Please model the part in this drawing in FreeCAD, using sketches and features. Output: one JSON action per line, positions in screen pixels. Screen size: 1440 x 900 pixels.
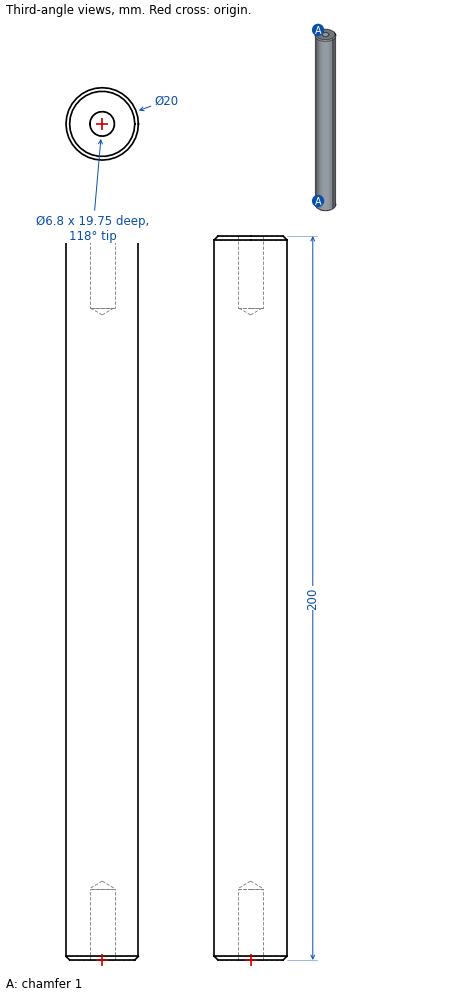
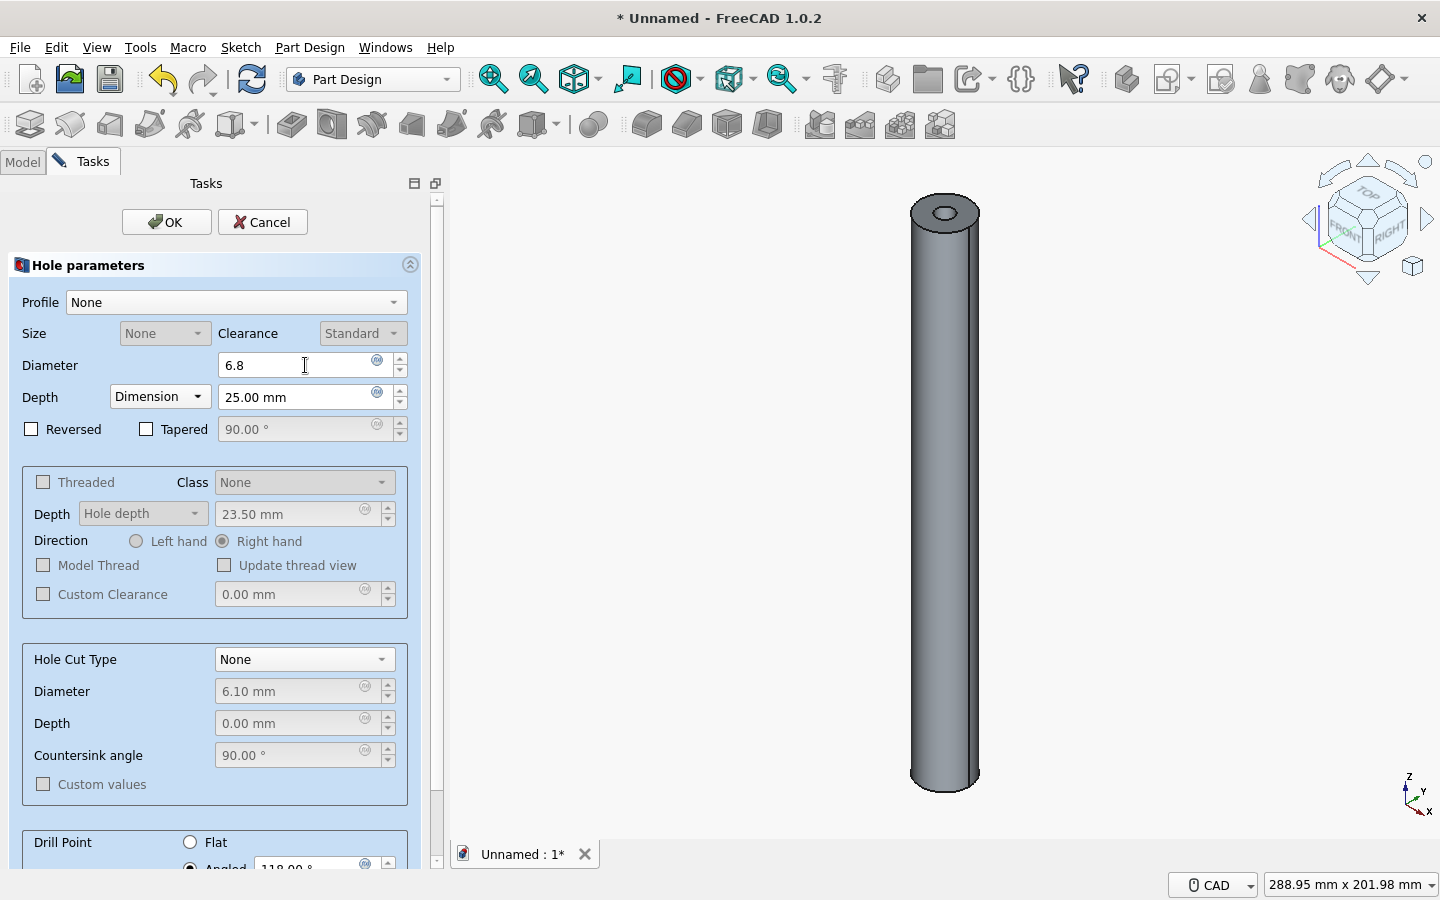
{"action": "triple_click", "coordinate": [305, 397]}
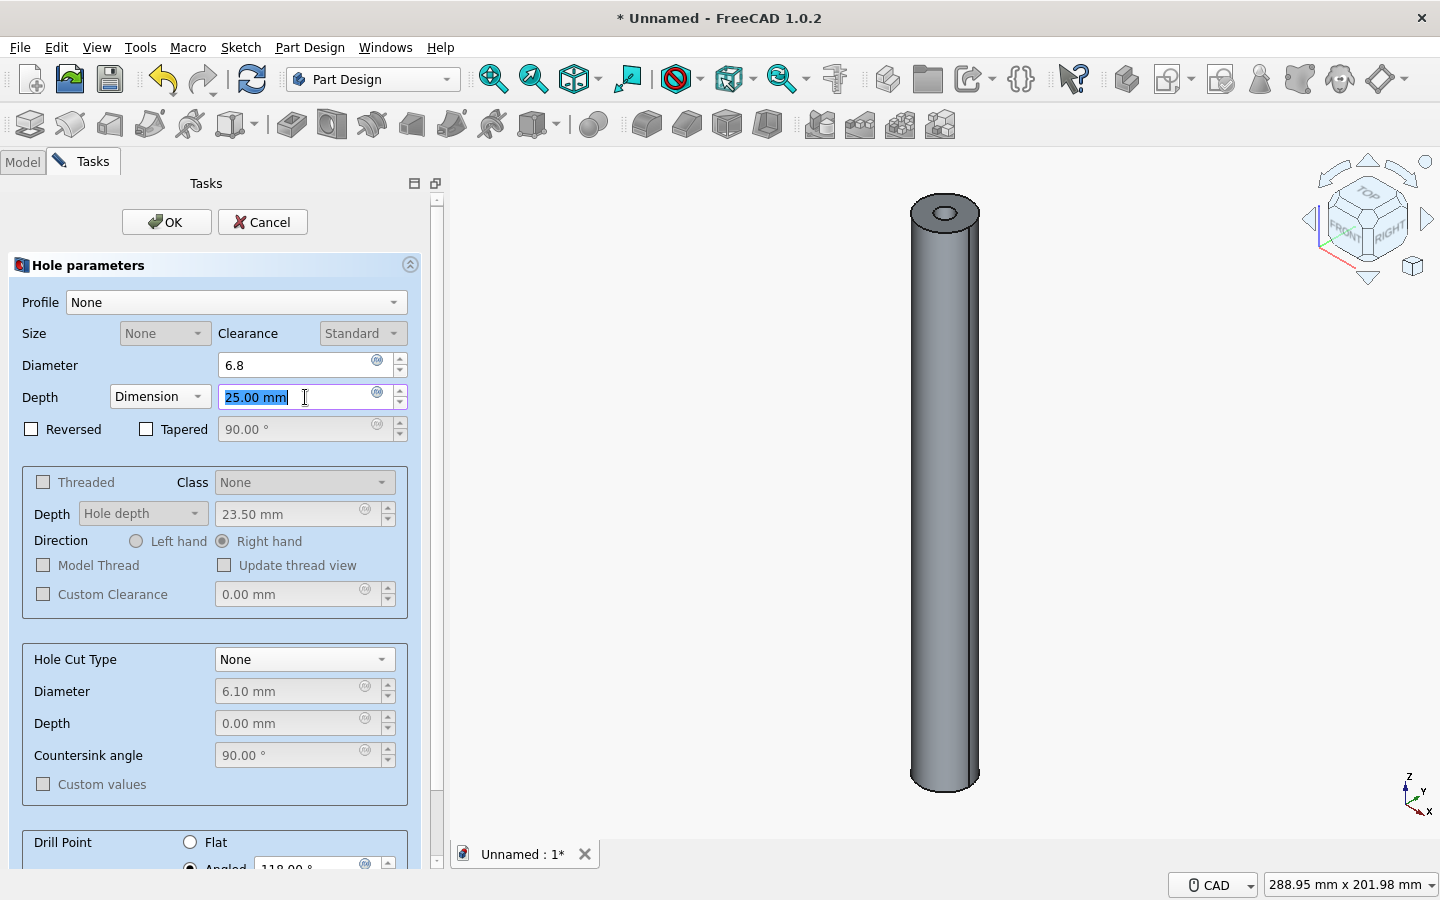
{"action": "type", "text": "19.75"}
{"action": "key", "text": "Tab"}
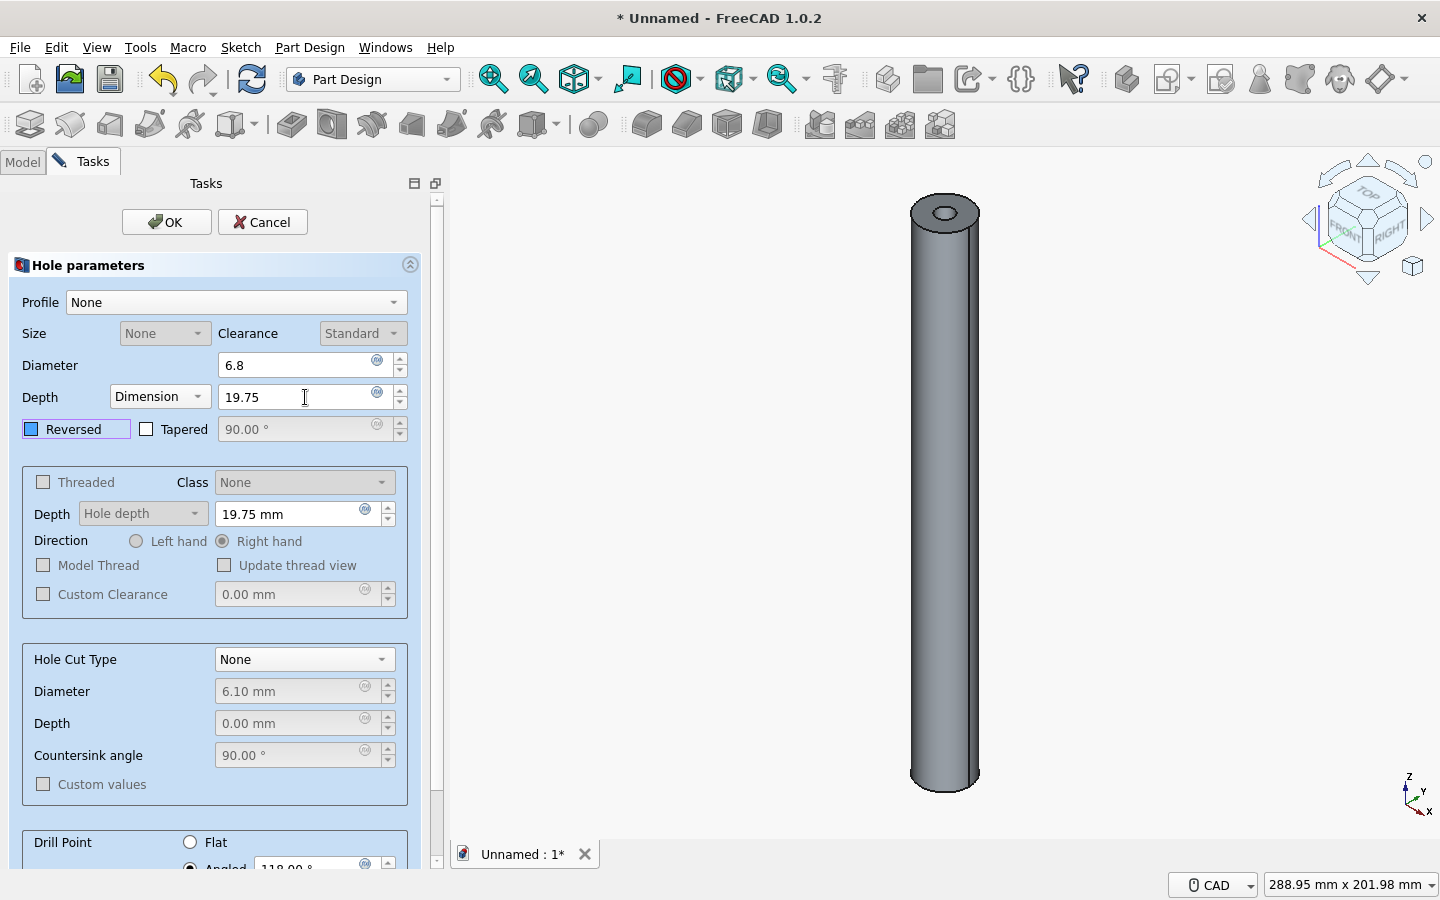
{"action": "left_click", "coordinate": [167, 222]}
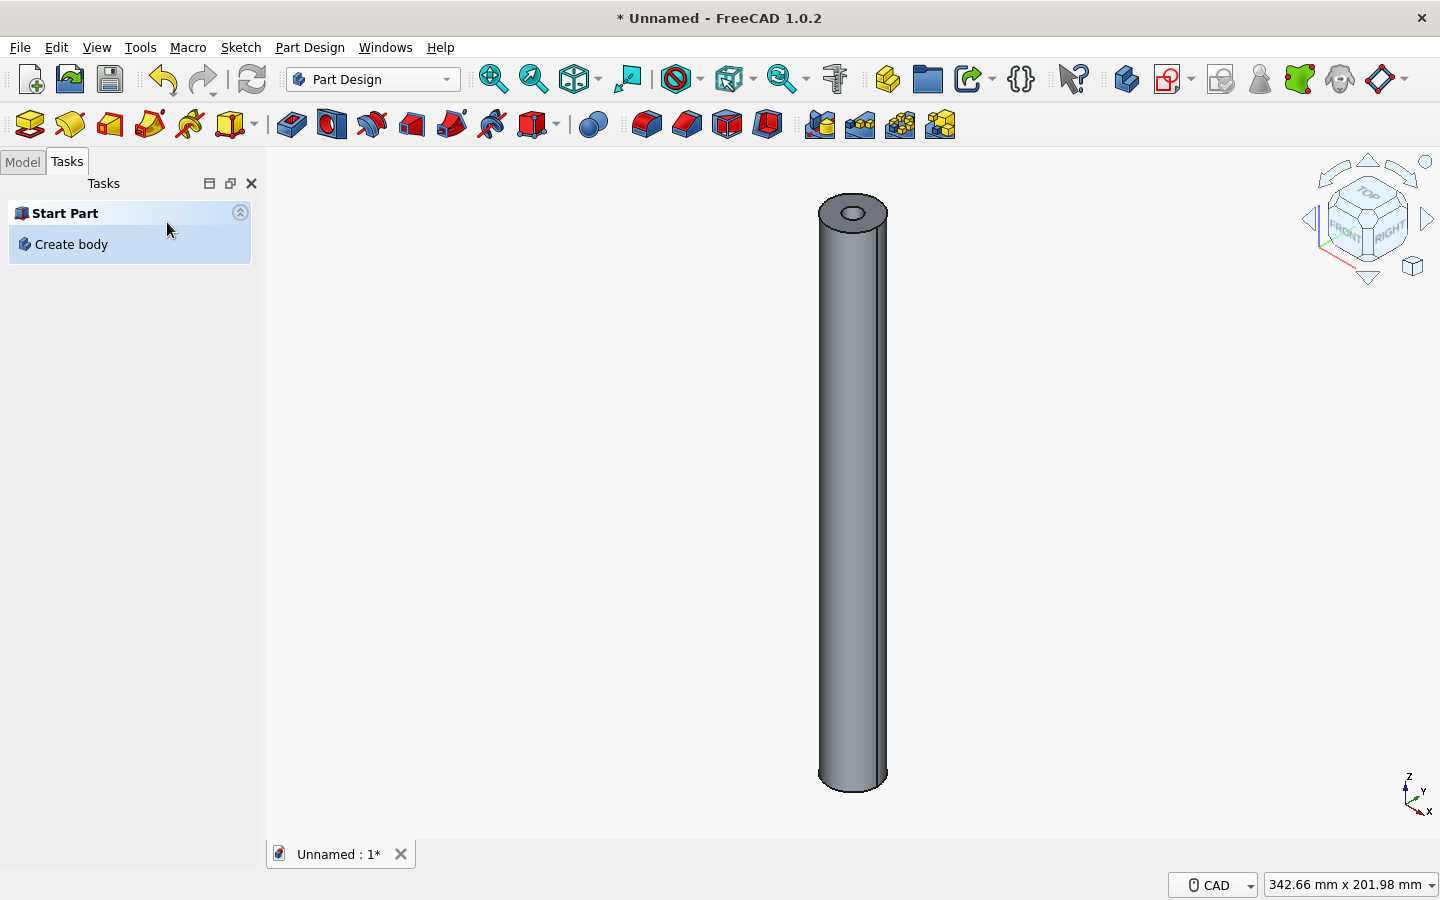
{"action": "left_click", "coordinate": [822, 221]}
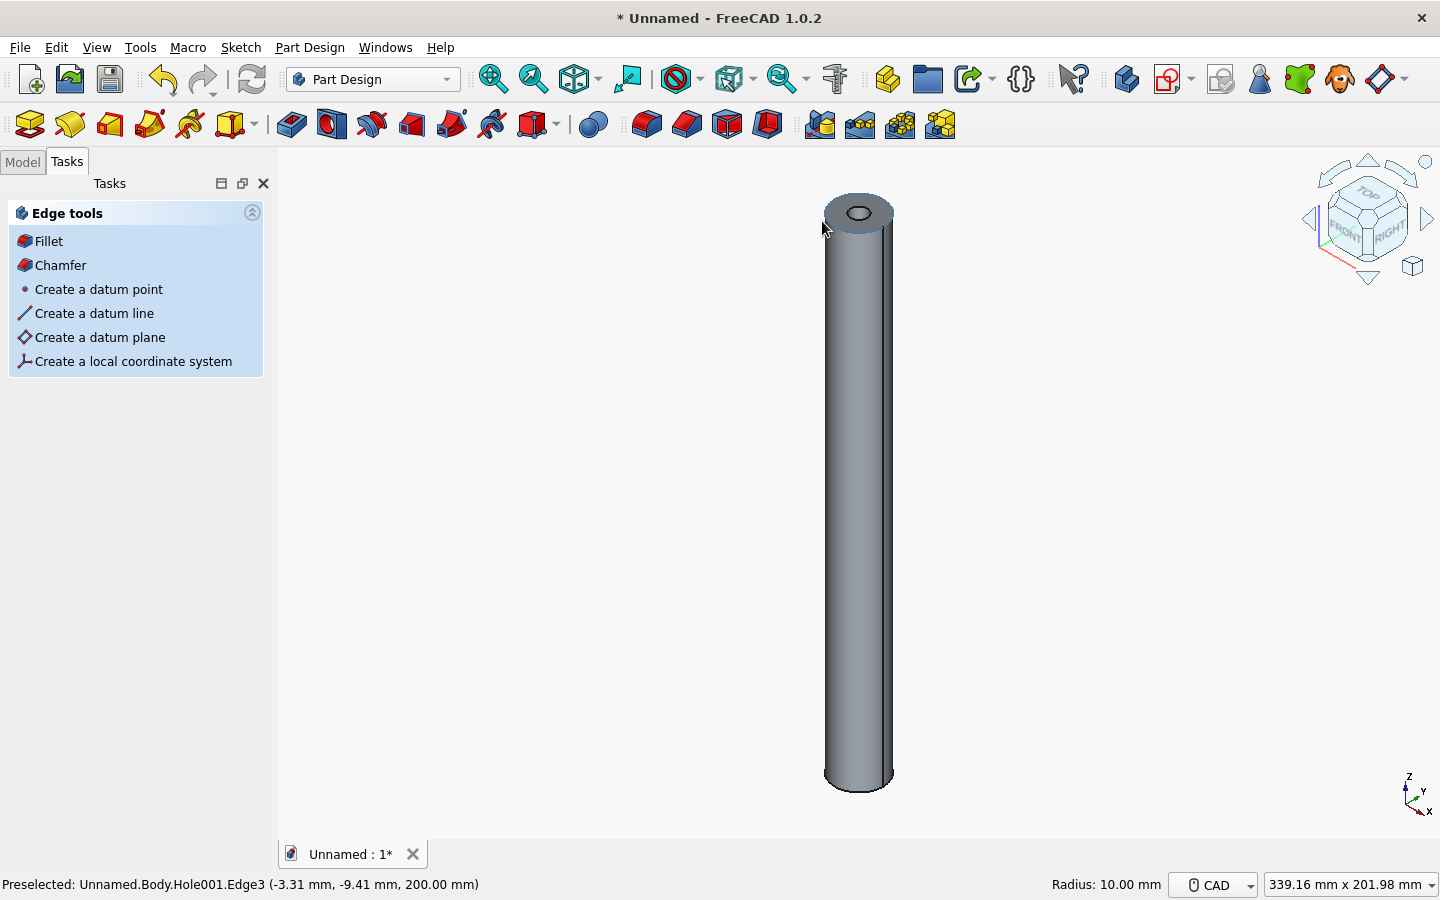
{"action": "key", "text": "2"}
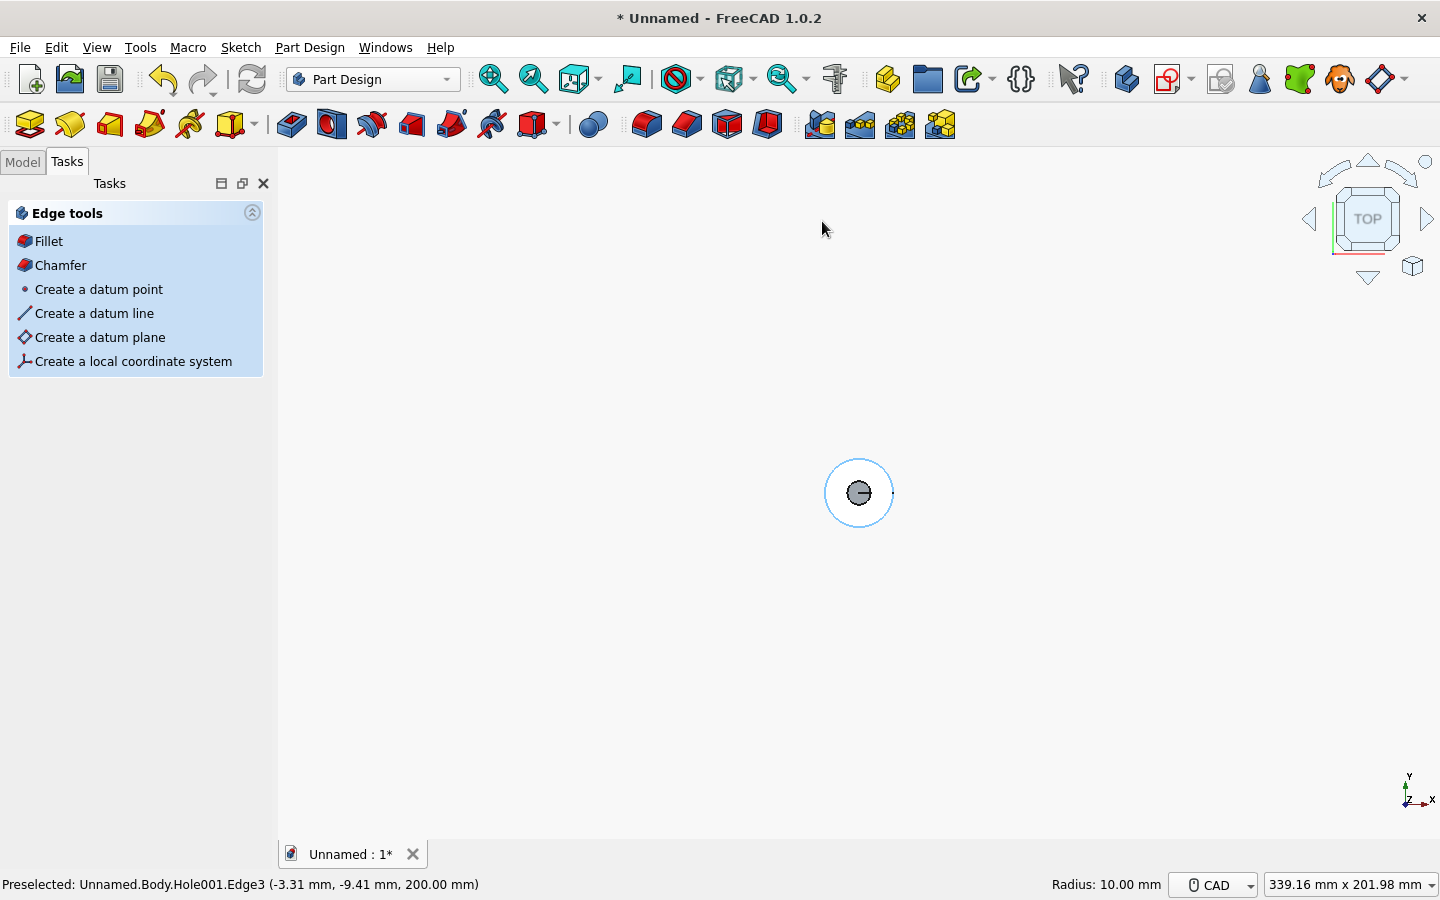
{"action": "key", "text": "v f"}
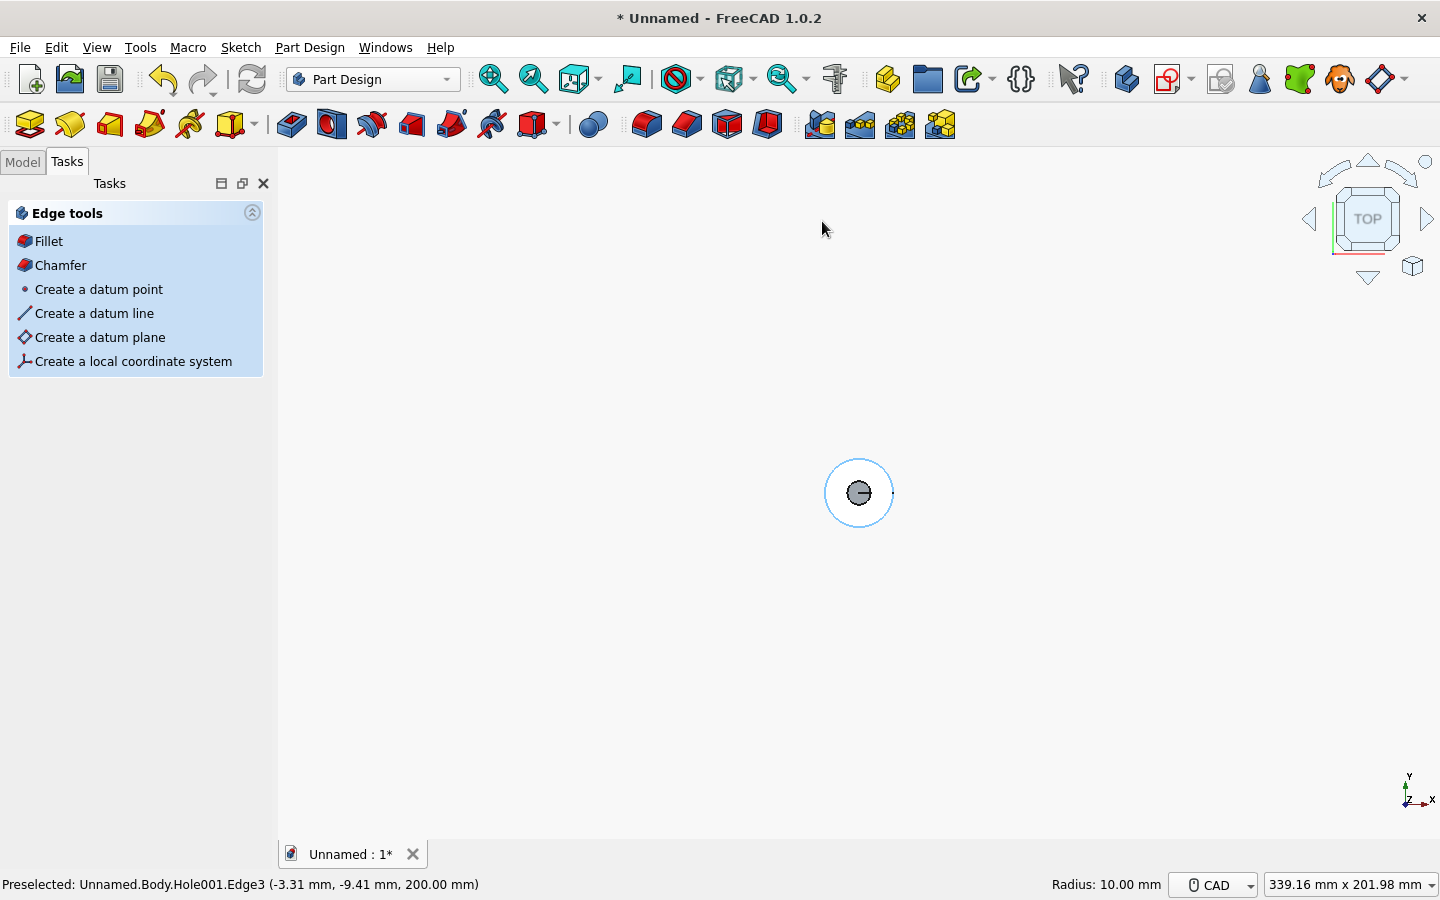
{"action": "key", "text": "0"}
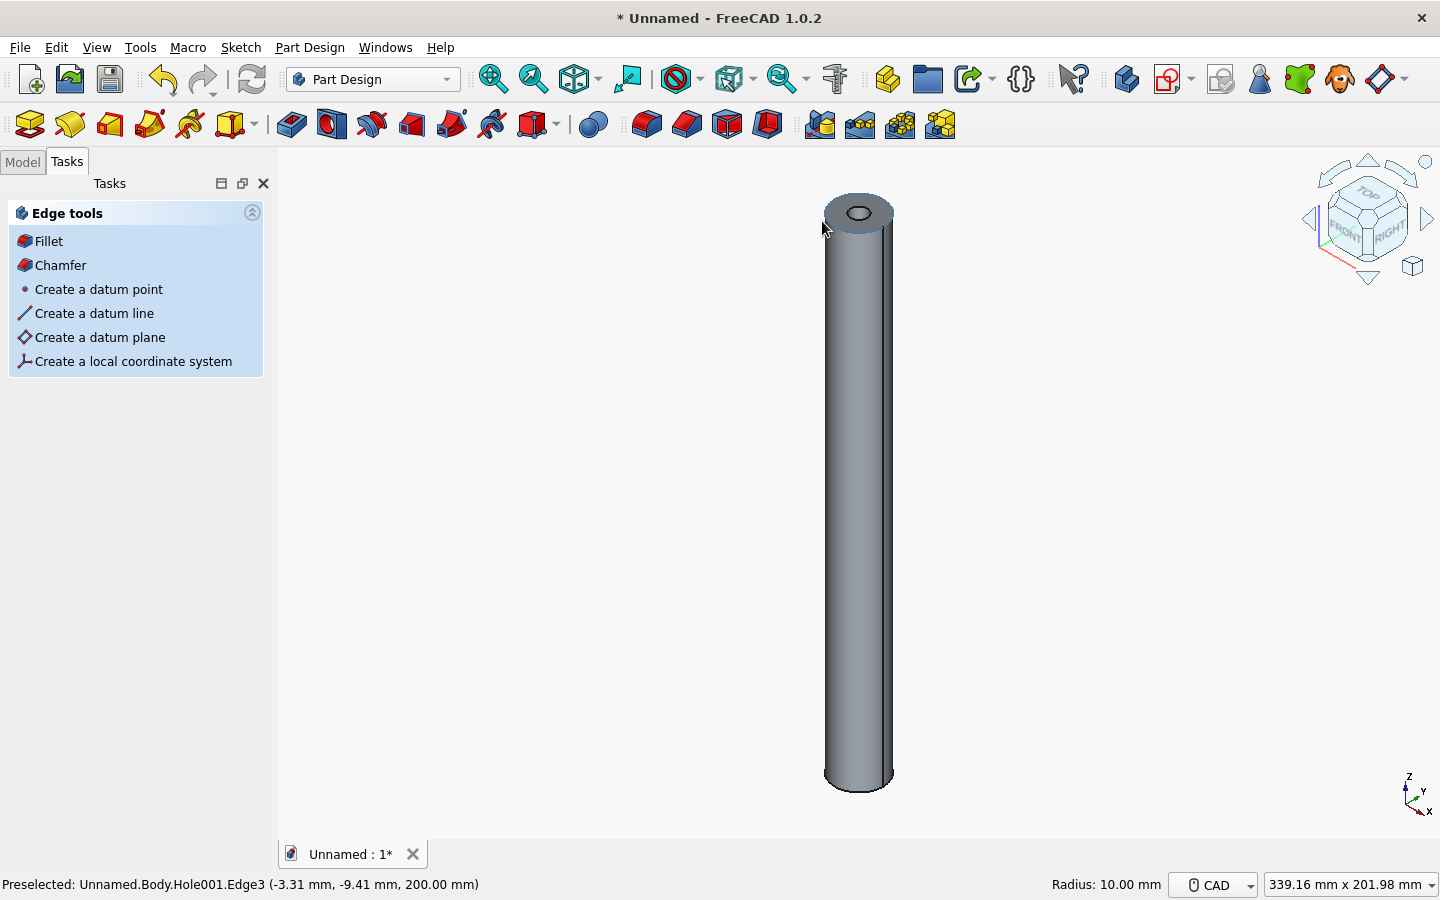
{"action": "key", "text": "1"}